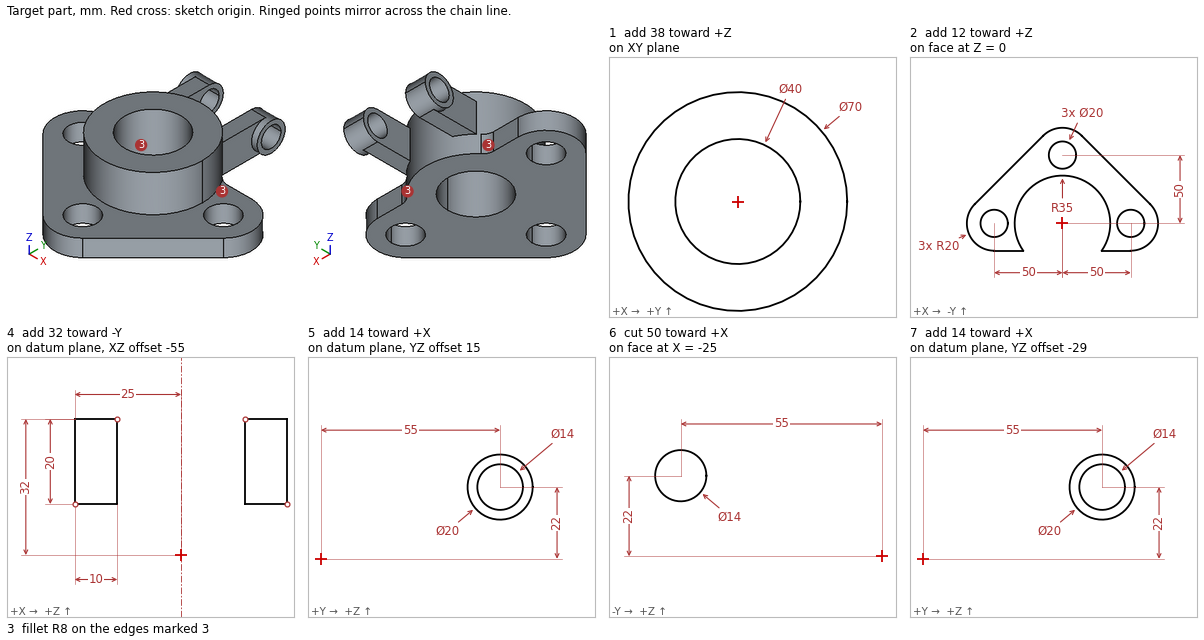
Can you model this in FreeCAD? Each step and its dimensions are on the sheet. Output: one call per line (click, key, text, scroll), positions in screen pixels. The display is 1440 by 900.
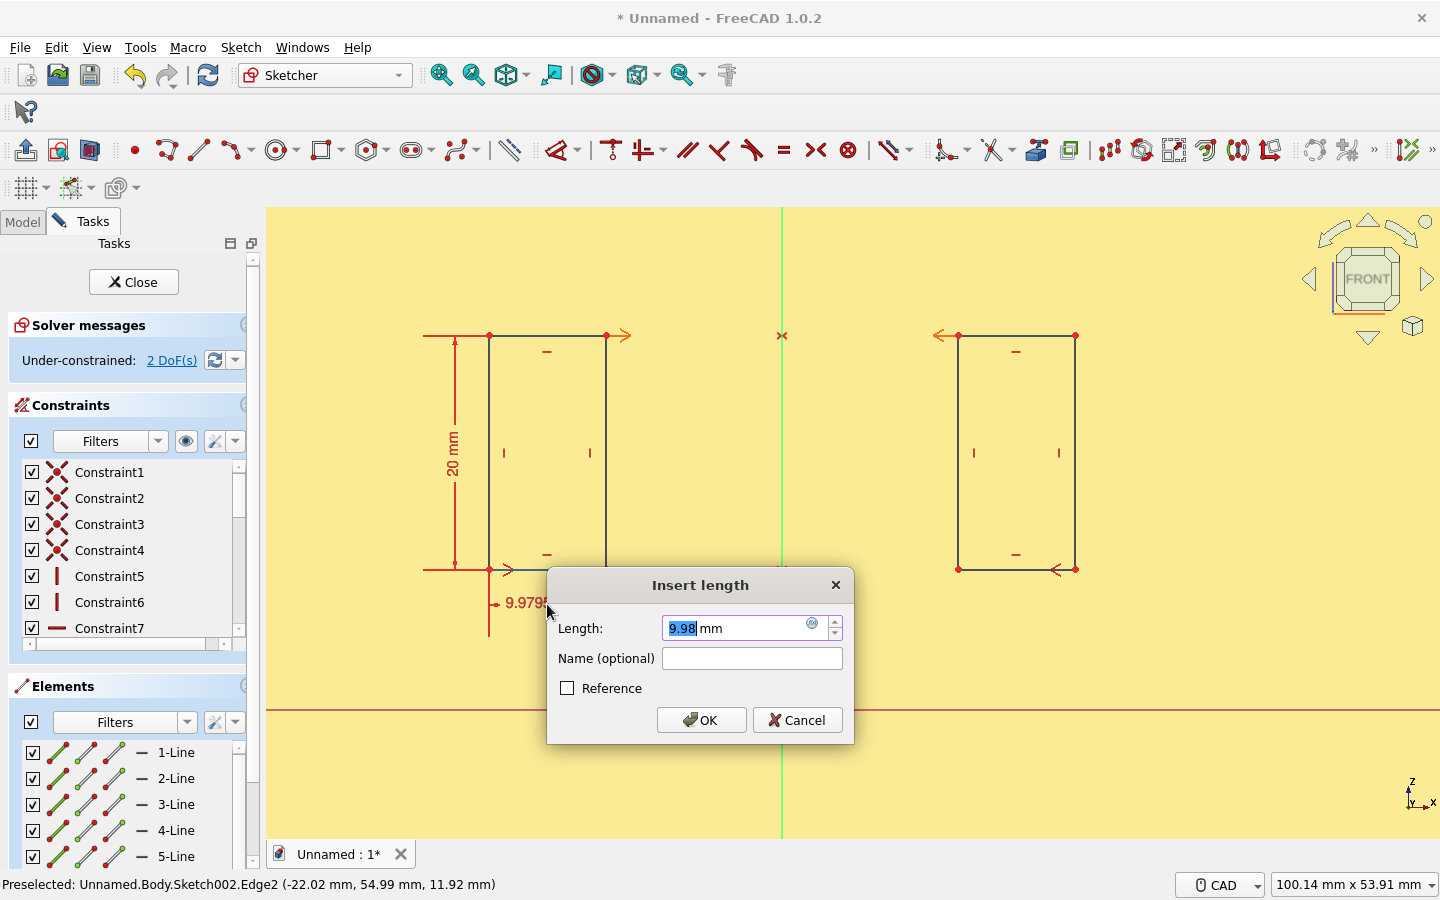
text(10)
key(Return)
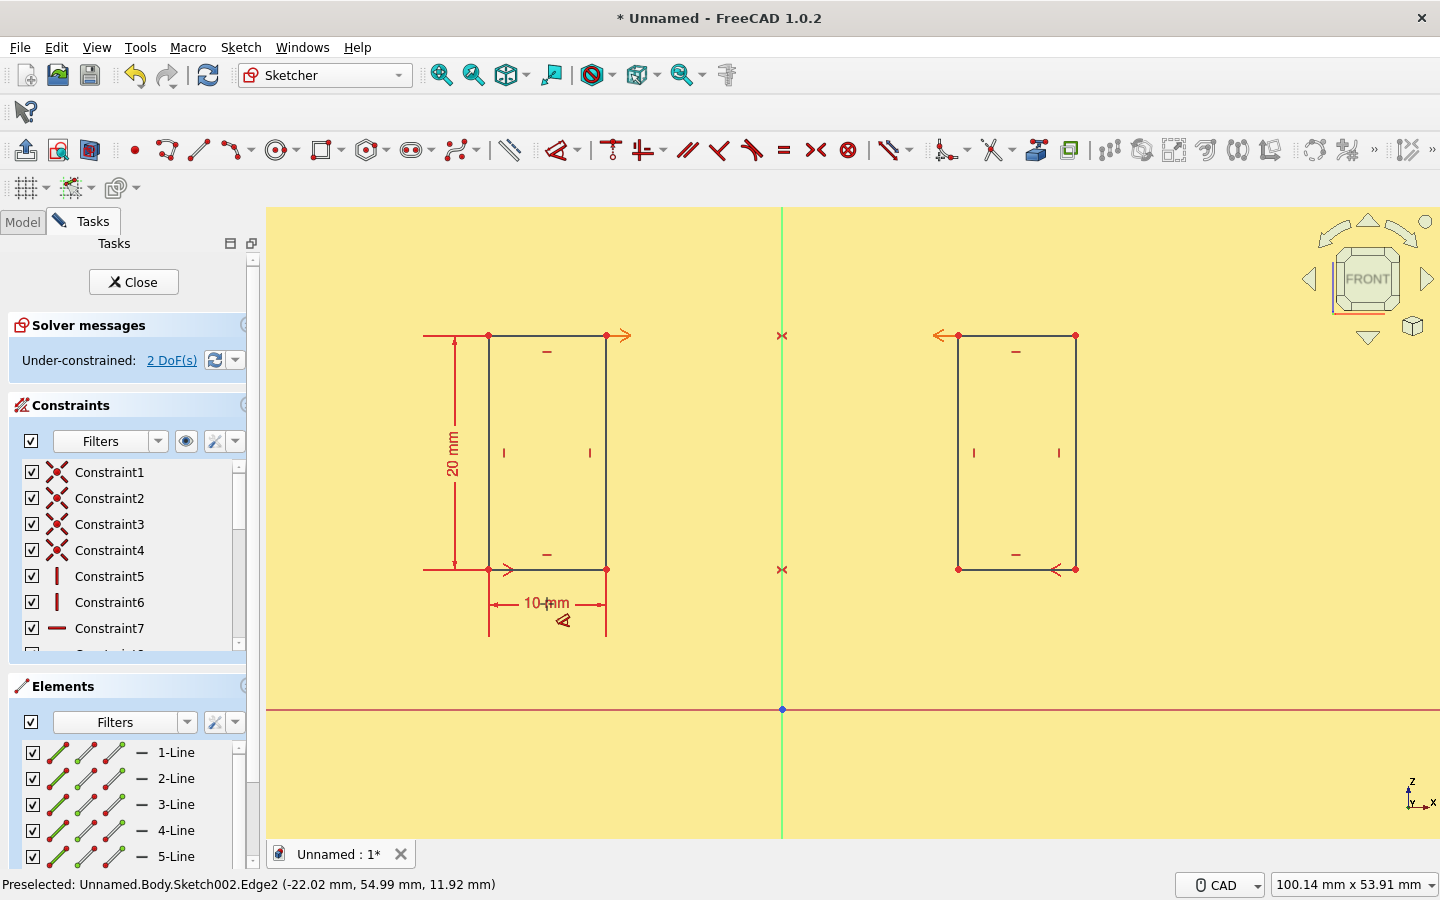
click(489, 336)
click(635, 744)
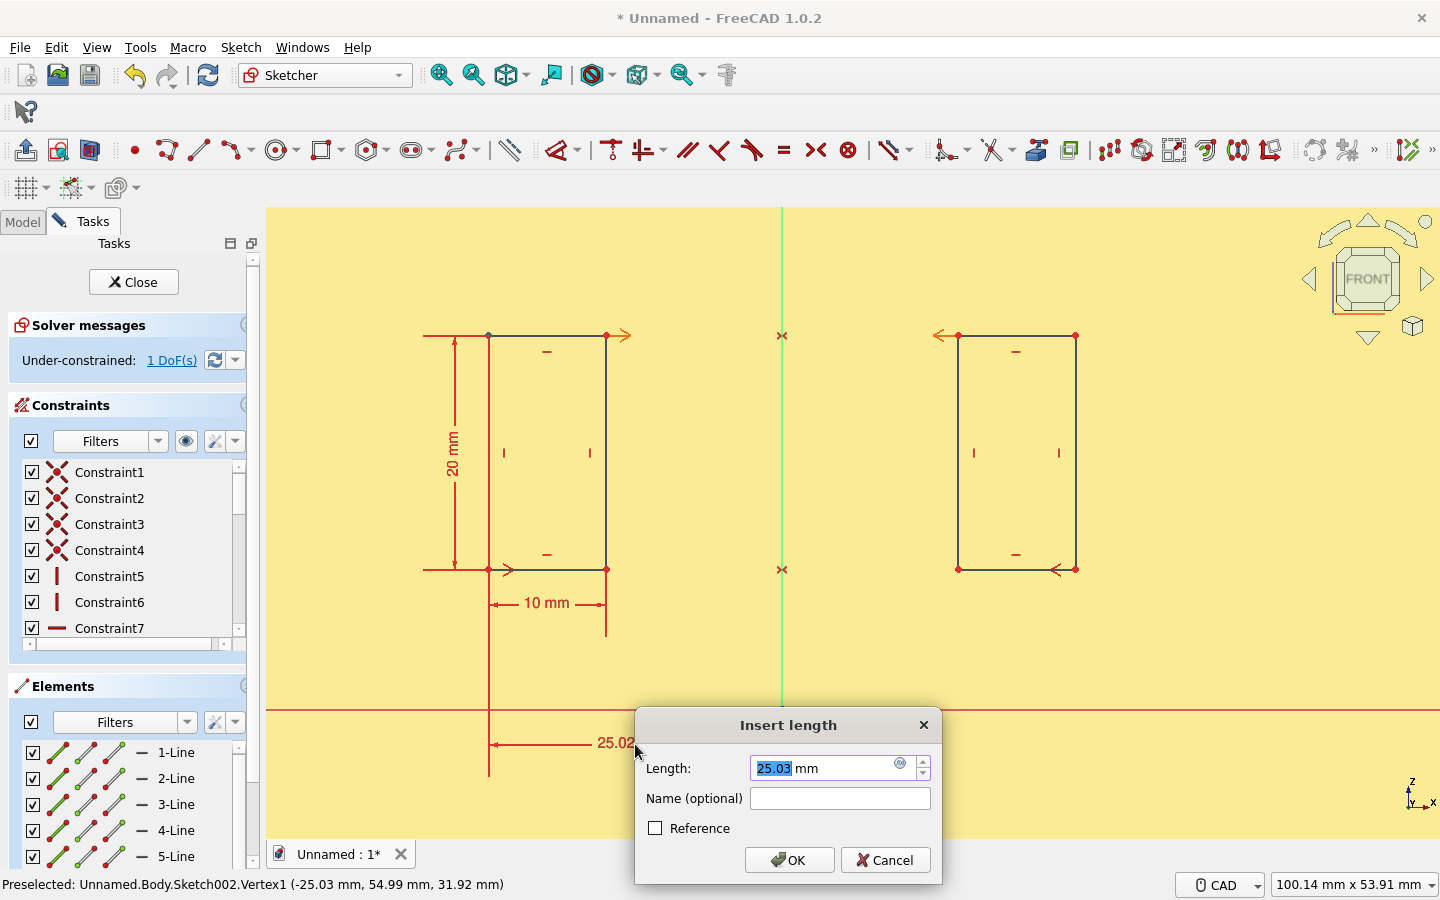
text(25)
key(Return)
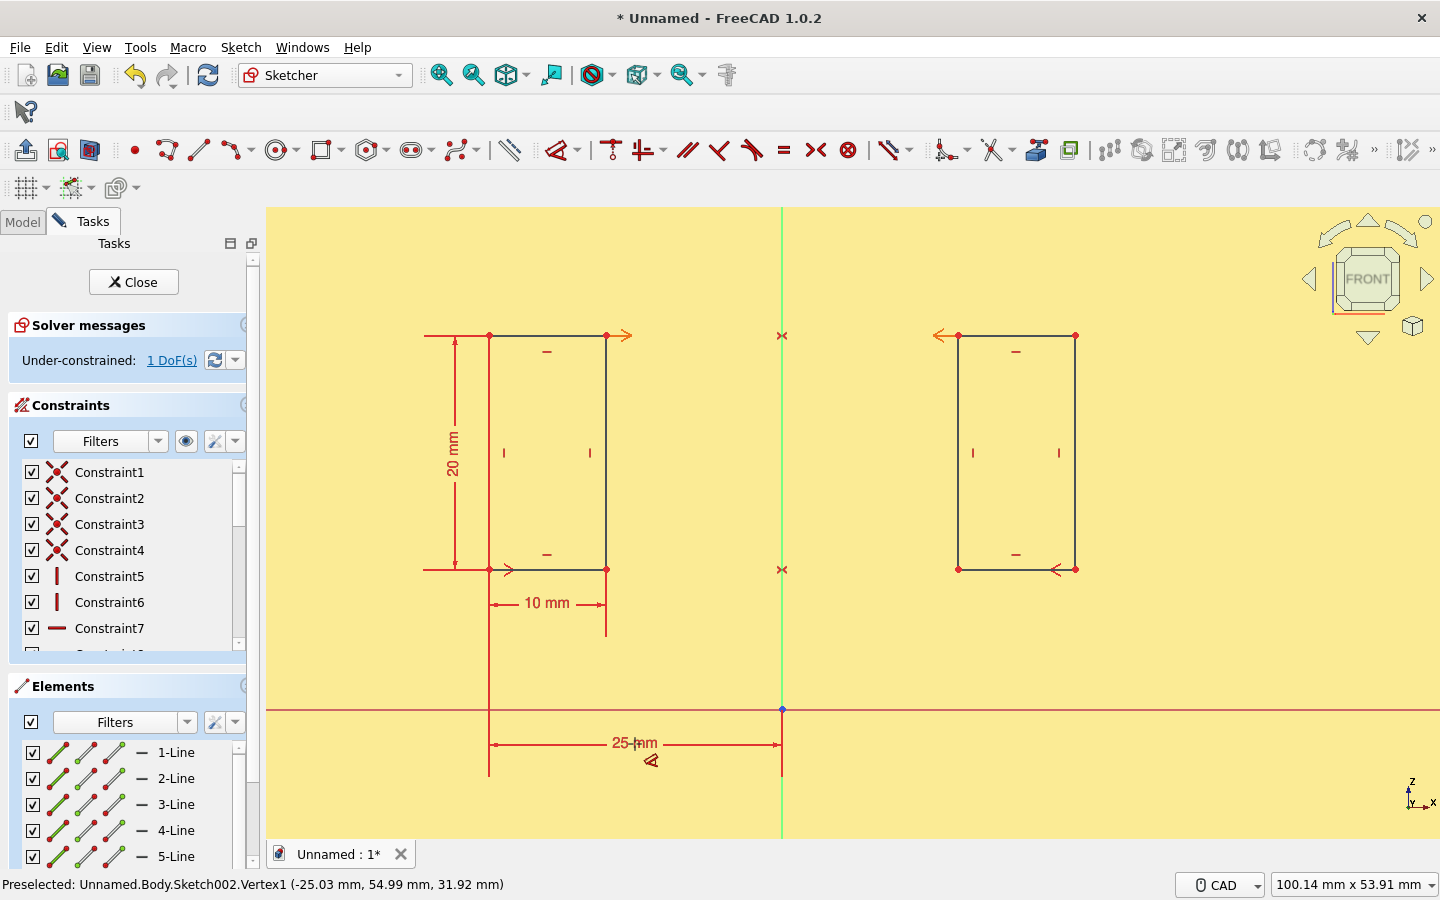
click(489, 336)
click(455, 523)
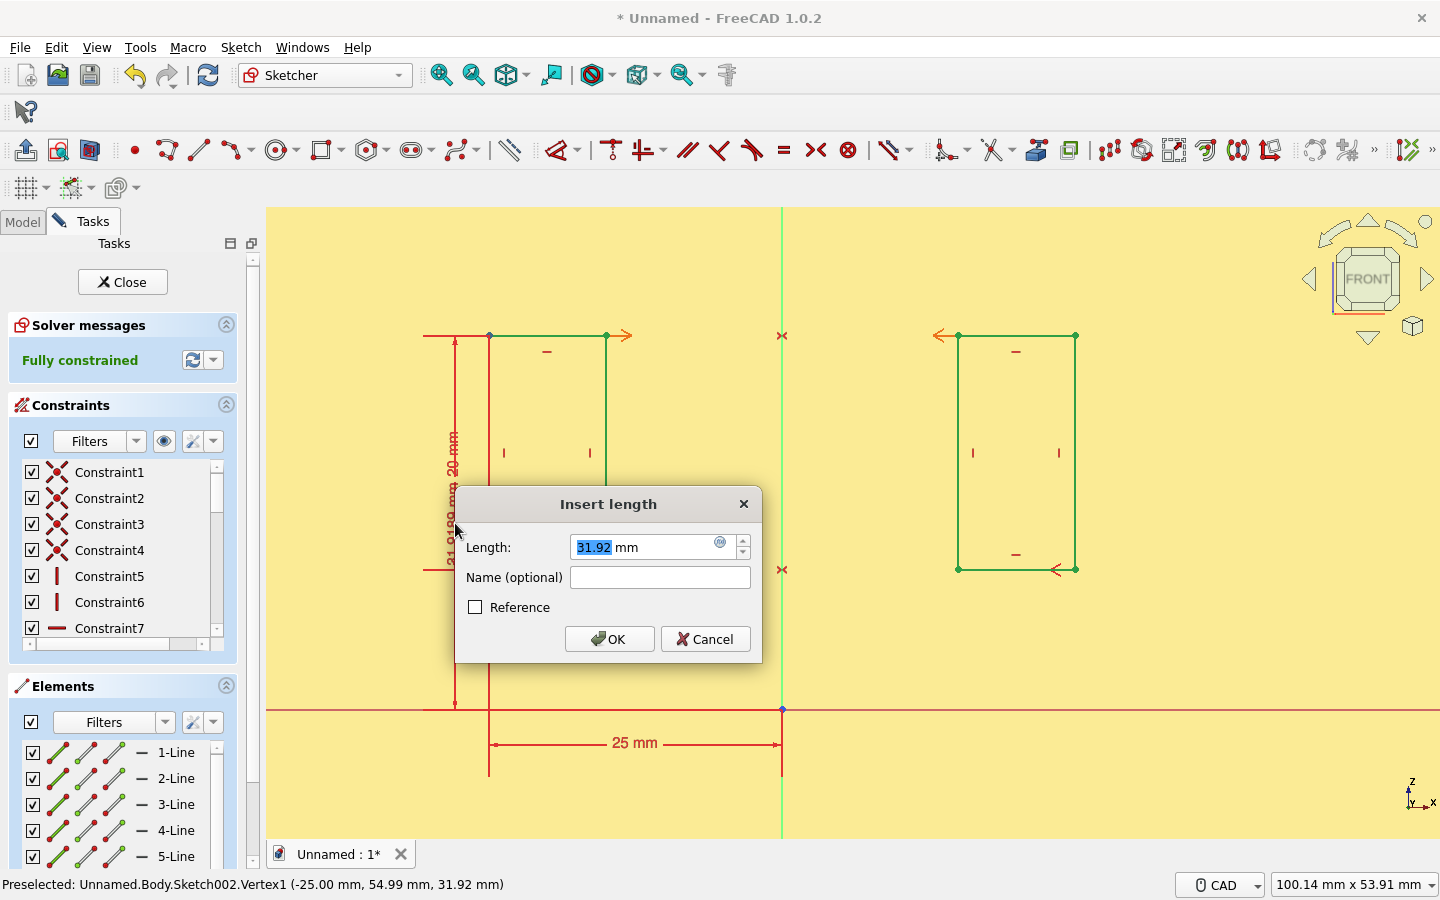
text(32)
key(Return)
key(Escape)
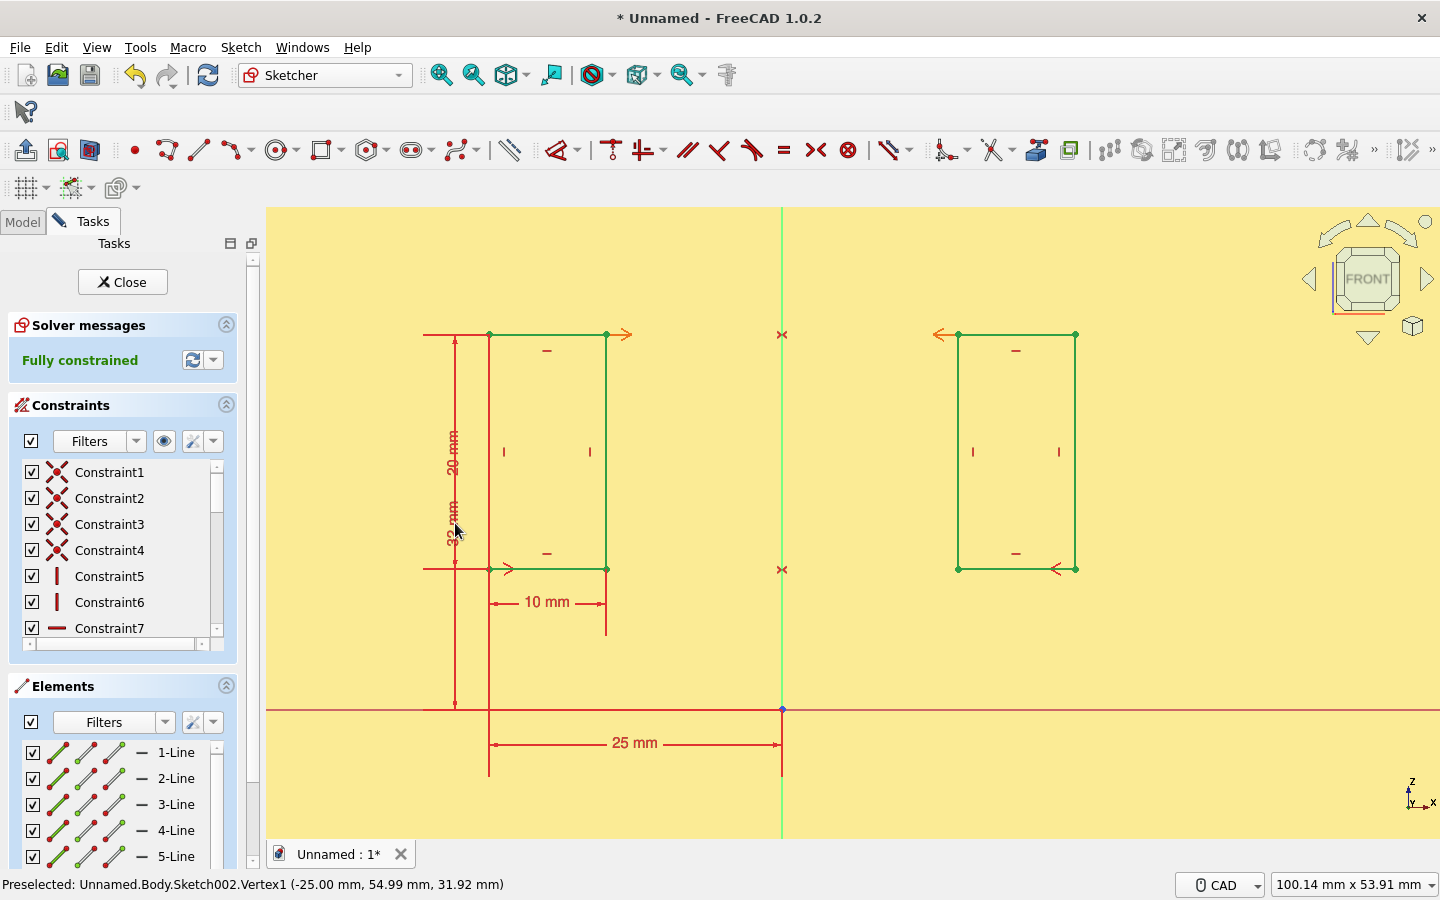
click(123, 282)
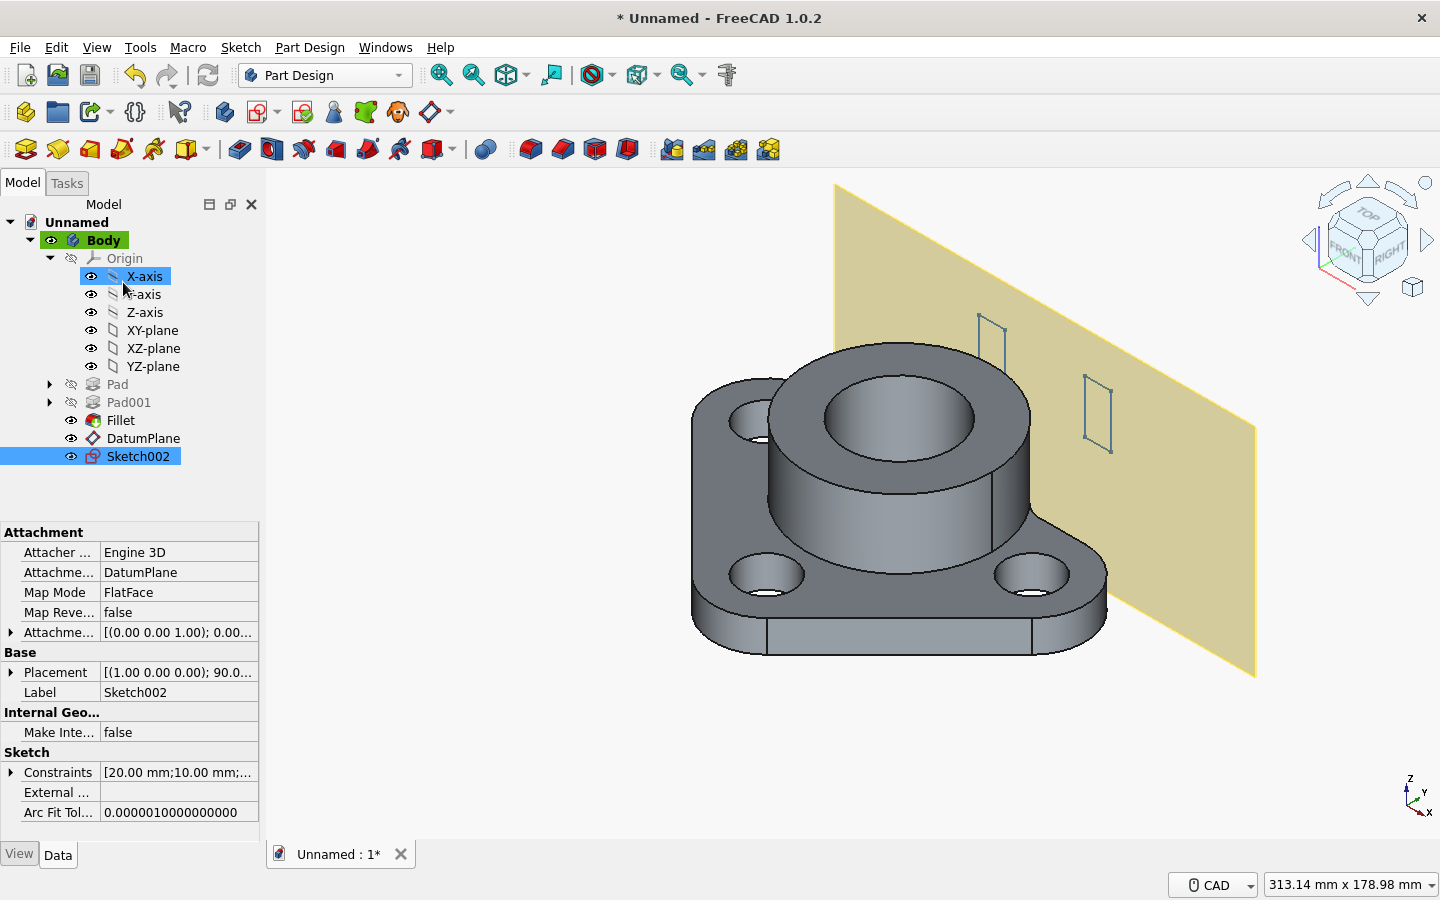
click(26, 150)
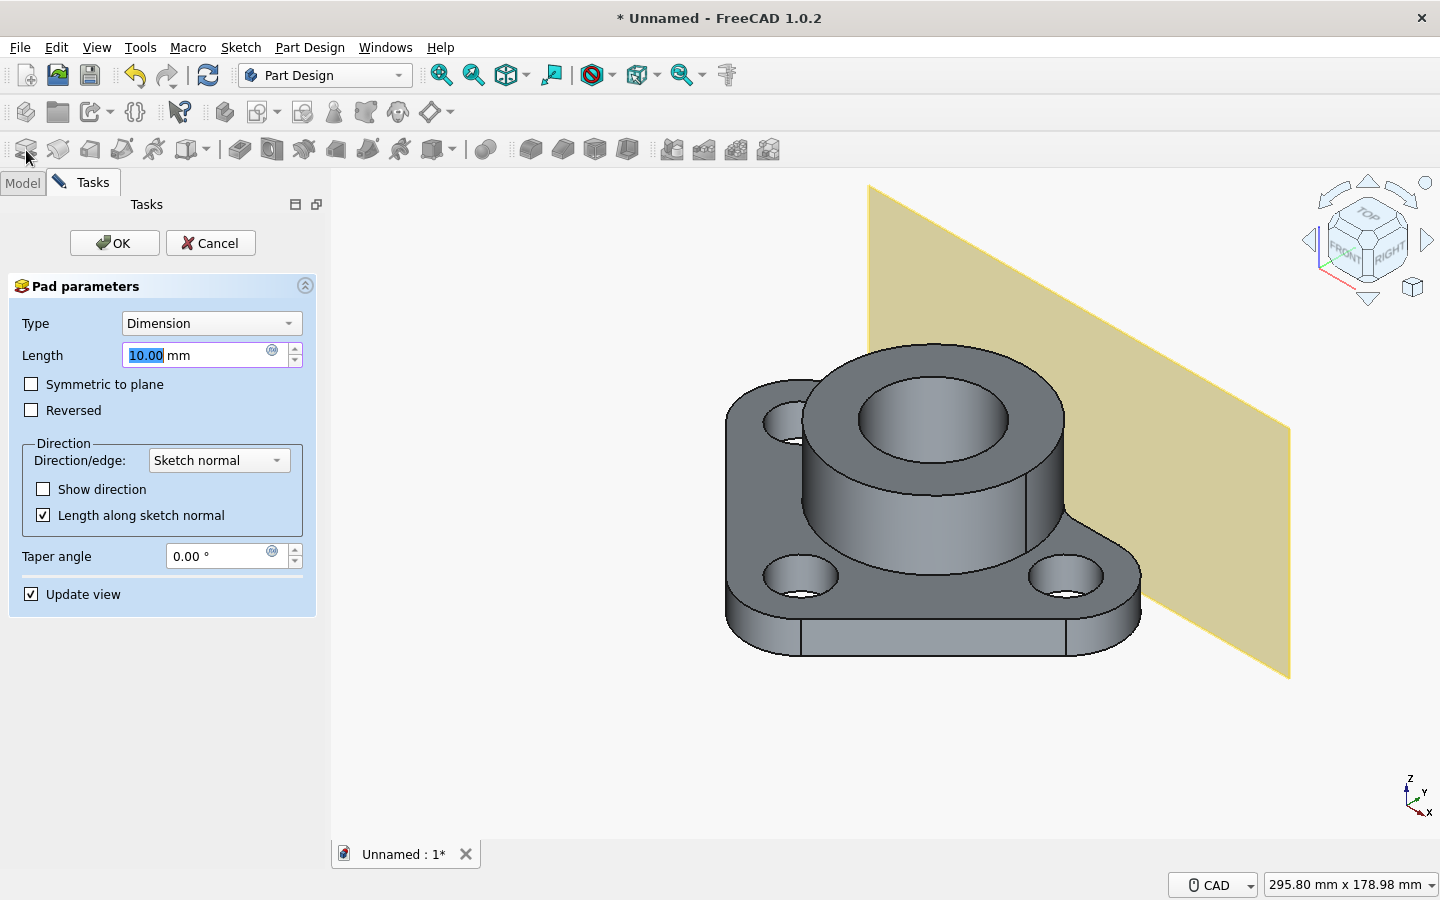
text(32)
key(Tab)